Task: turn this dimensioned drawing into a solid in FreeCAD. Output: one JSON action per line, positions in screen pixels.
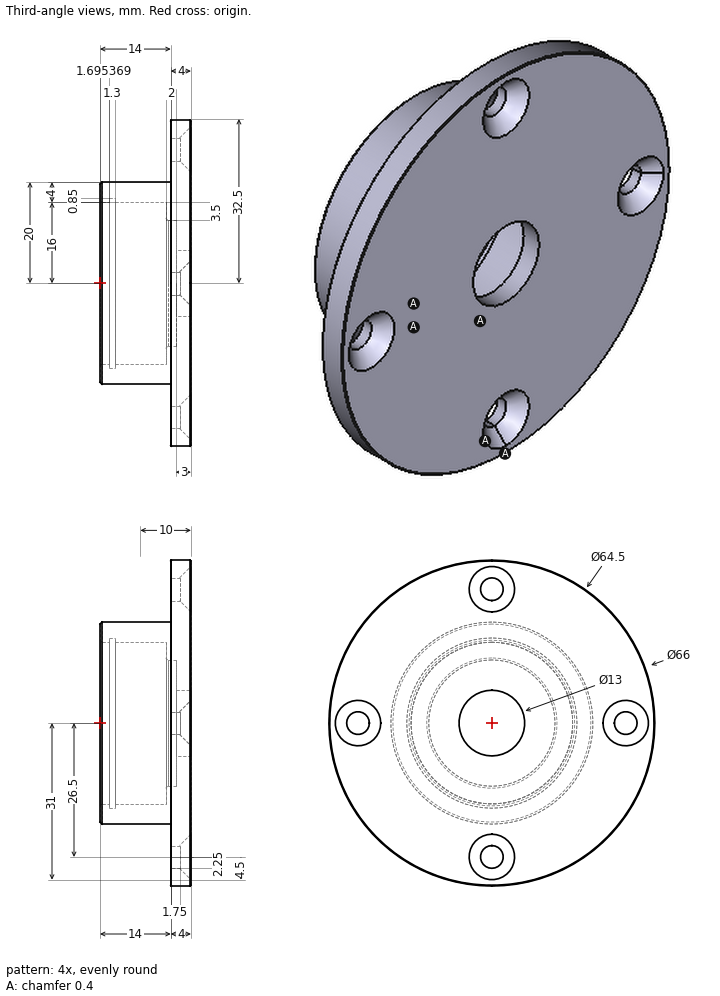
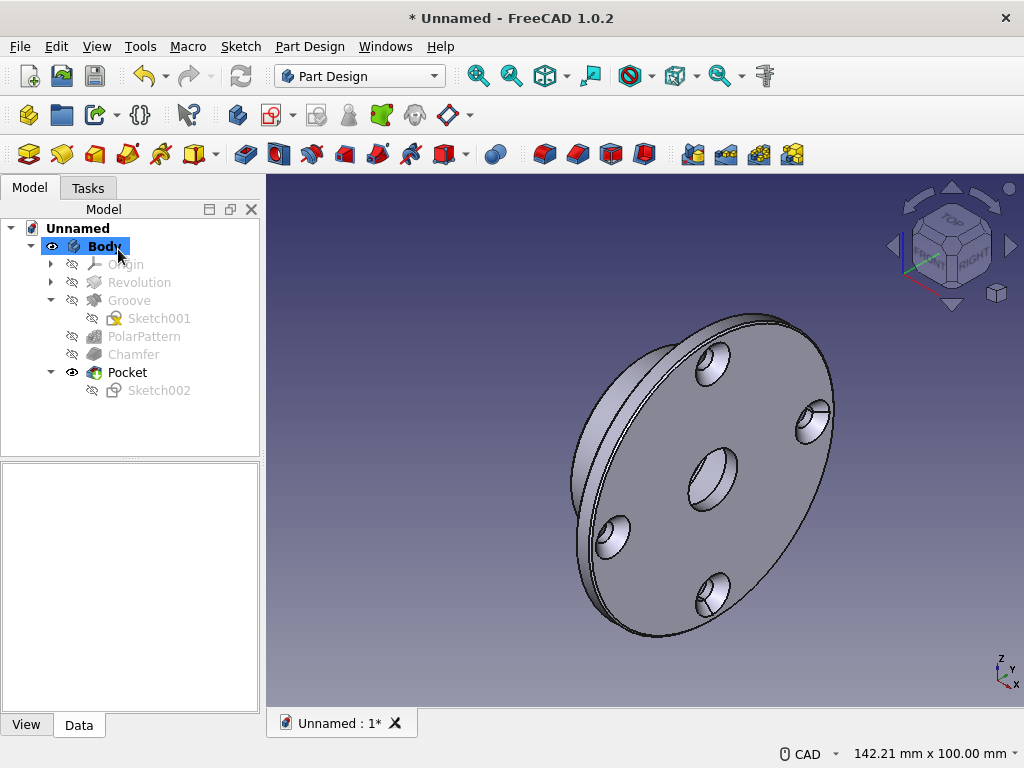
{"action": "left_click", "coordinate": [782, 399]}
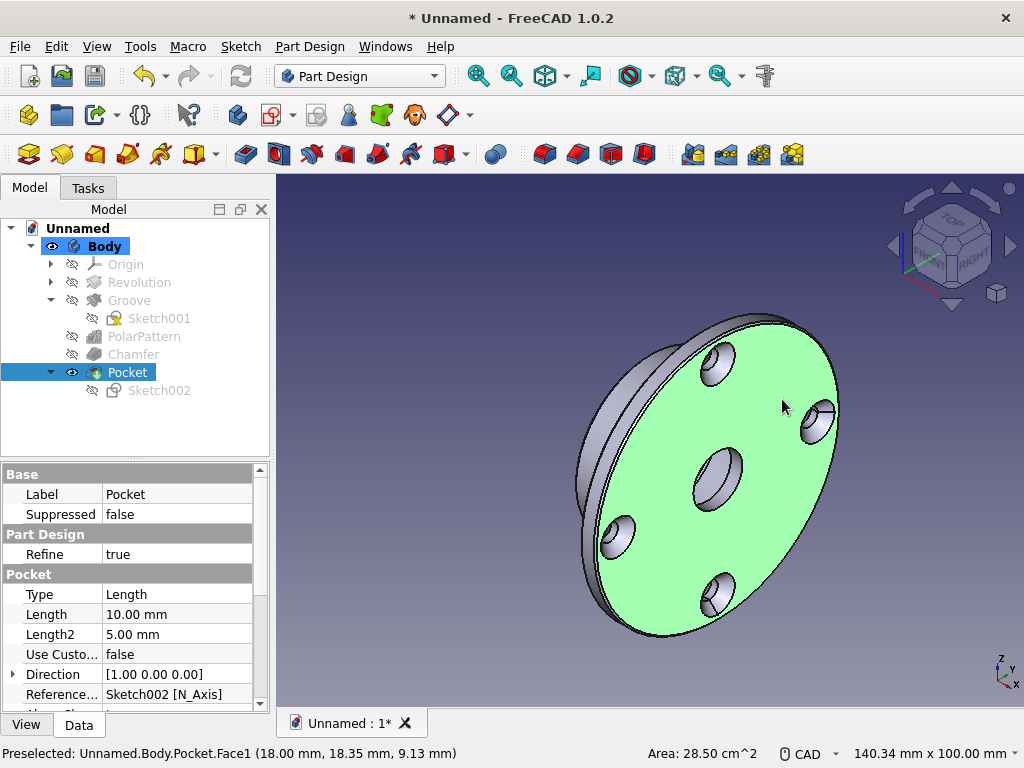
{"action": "left_click", "coordinate": [270, 116]}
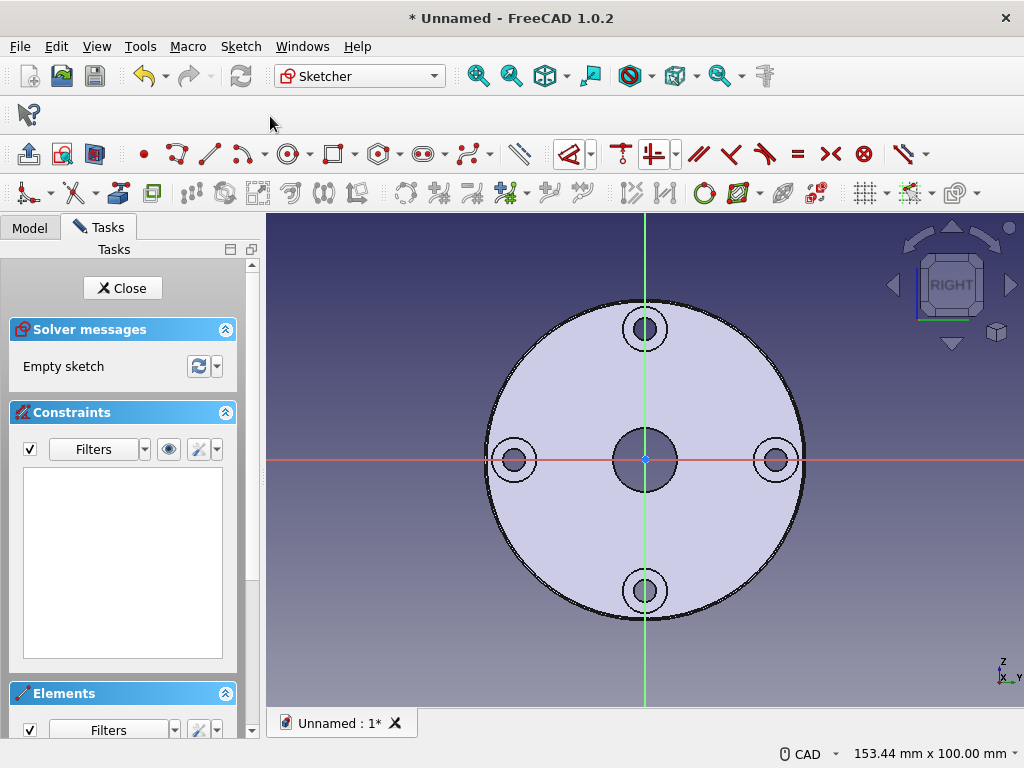
{"action": "left_click", "coordinate": [288, 154]}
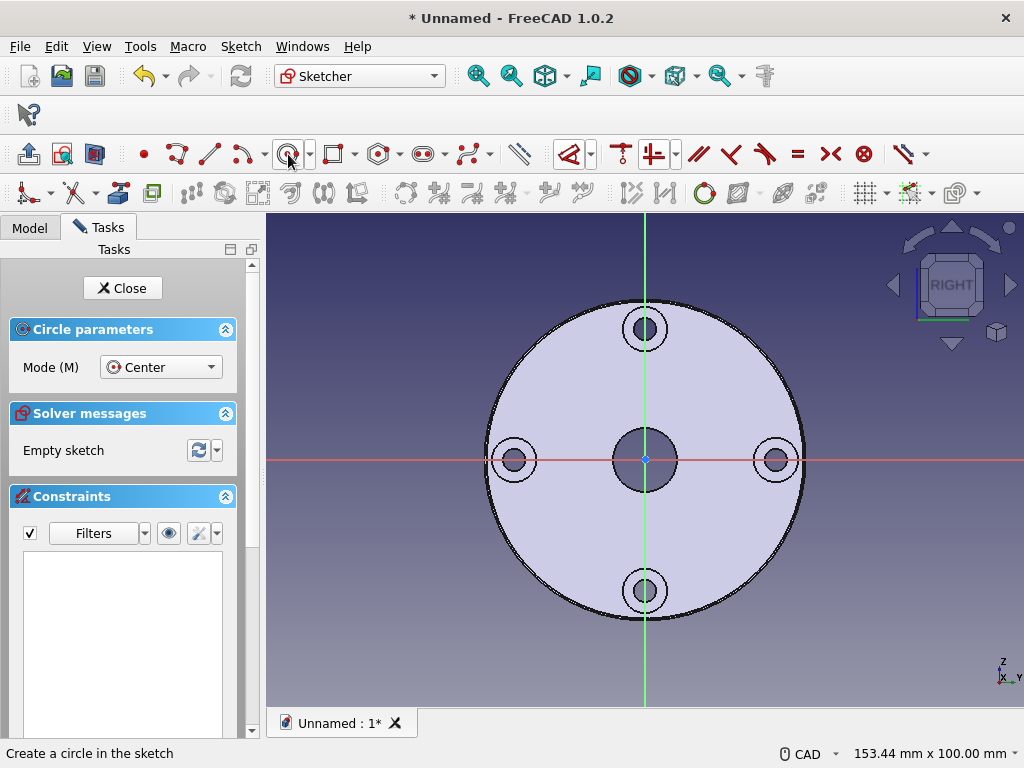
{"action": "left_click", "coordinate": [645, 460]}
{"action": "mouse_move", "coordinate": [760, 345]}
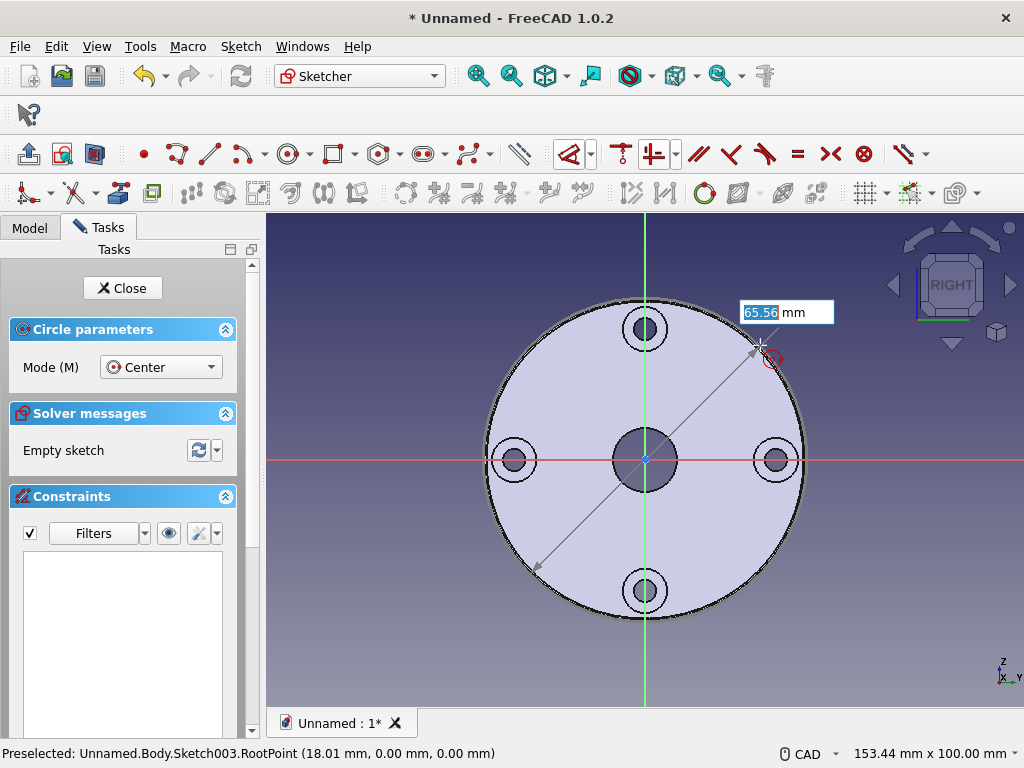
{"action": "type", "text": "66"}
{"action": "key", "text": "Return"}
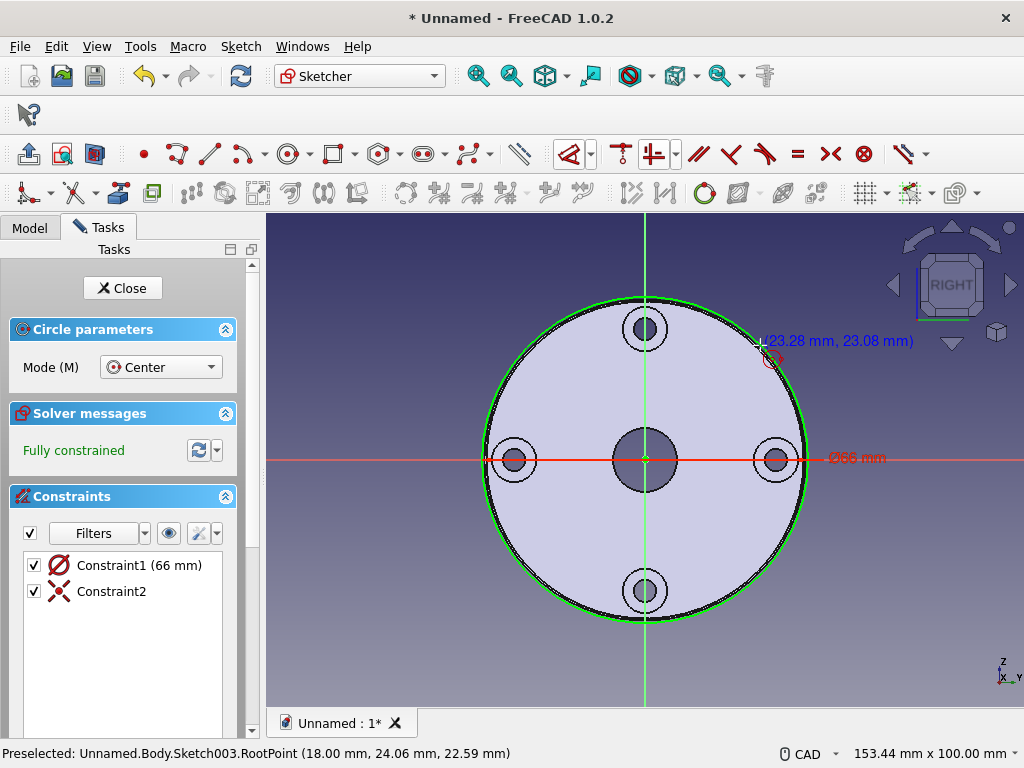
{"action": "left_click", "coordinate": [645, 460]}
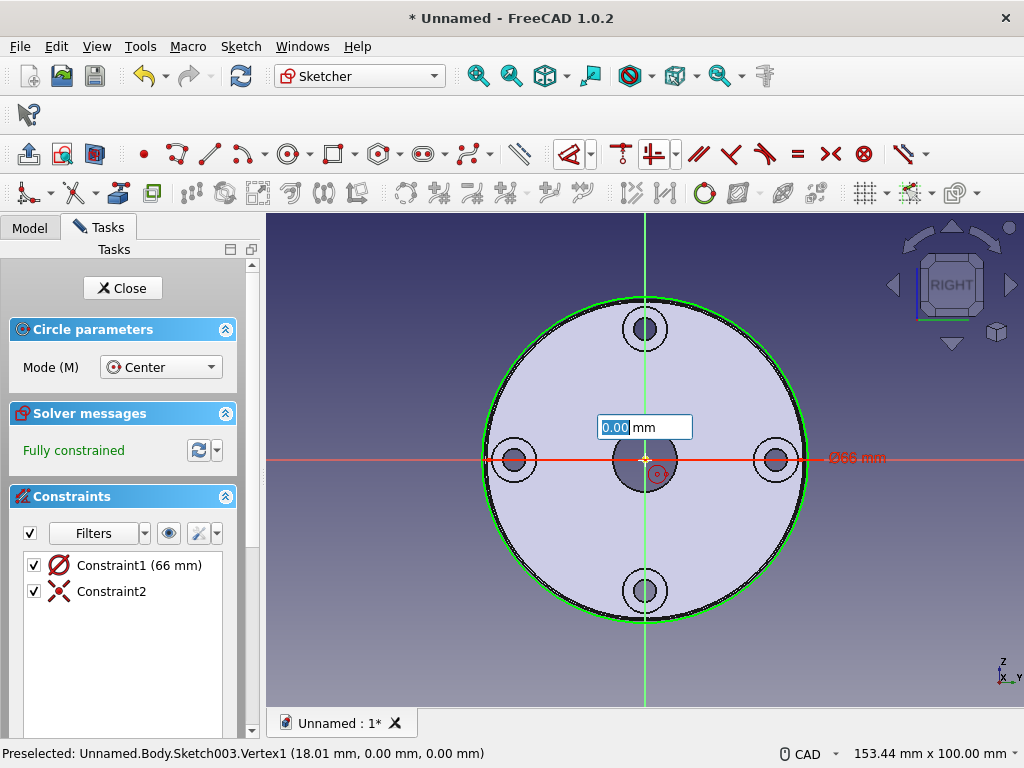
{"action": "scroll", "coordinate": [758, 347], "scroll_direction": "up", "scroll_amount": 8}
{"action": "mouse_move", "coordinate": [754, 348]}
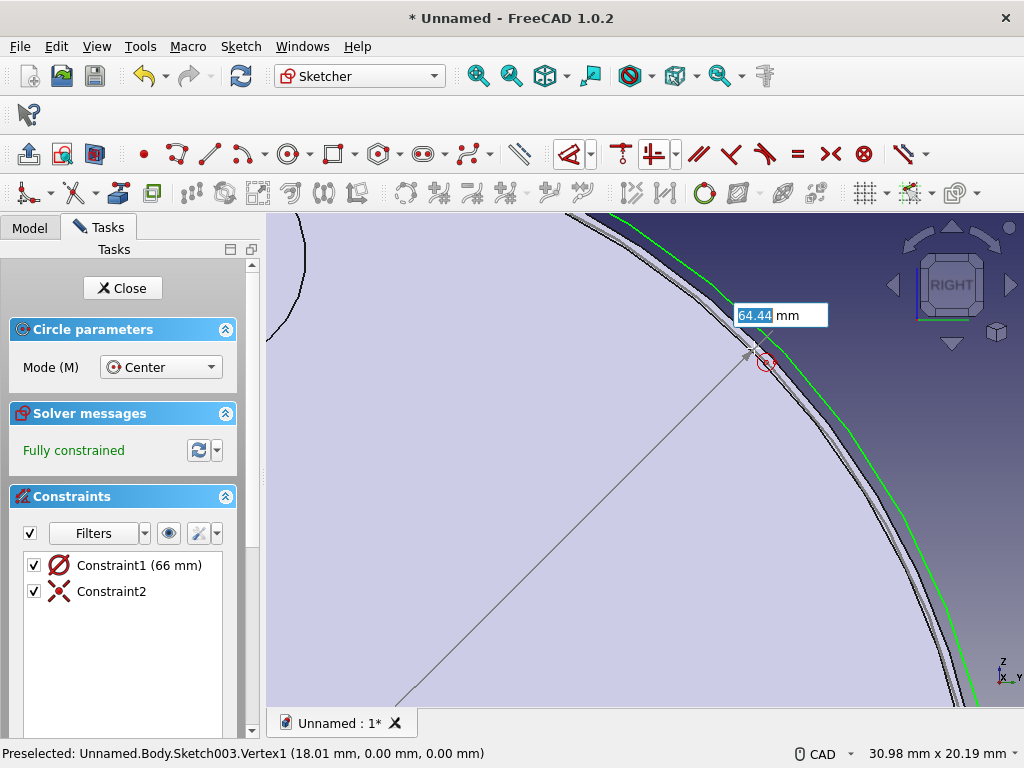
{"action": "type", "text": "64.5"}
{"action": "key", "text": "Return"}
{"action": "key", "text": "Escape"}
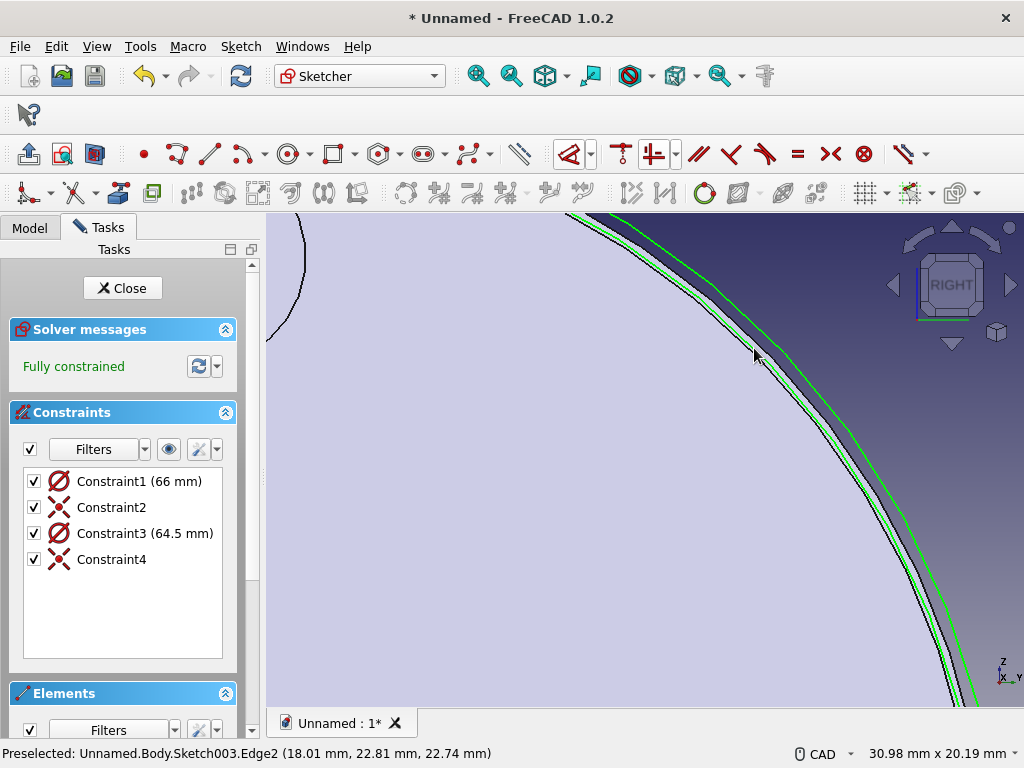
{"action": "left_click", "coordinate": [123, 288]}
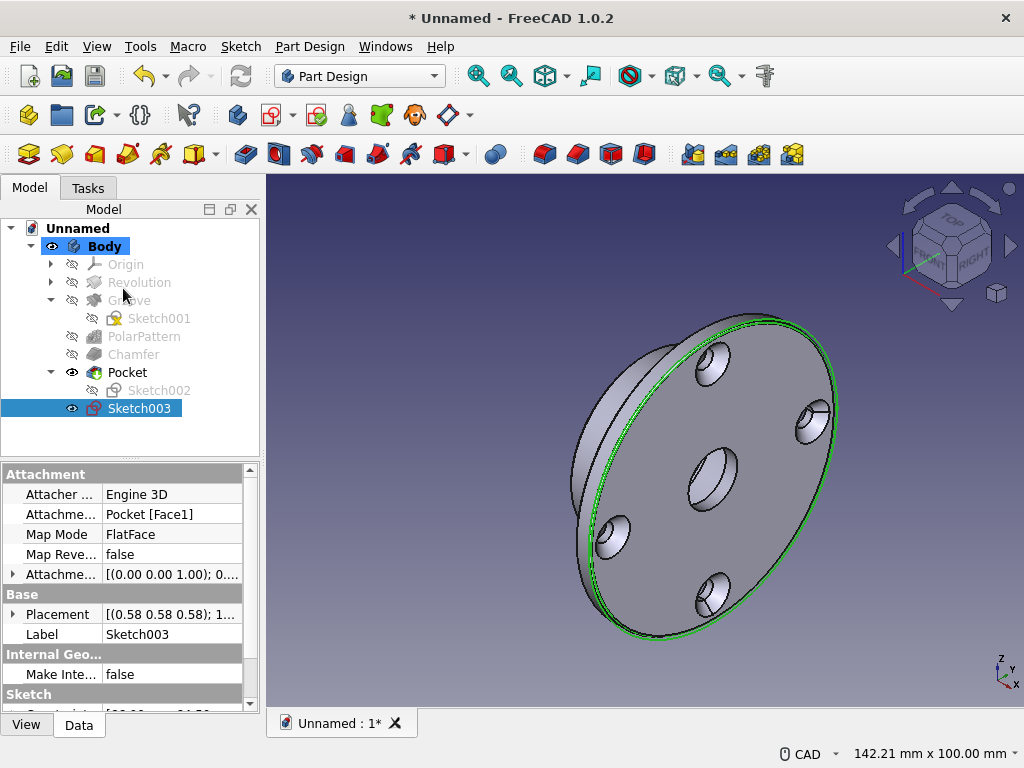
{"action": "left_click", "coordinate": [246, 154]}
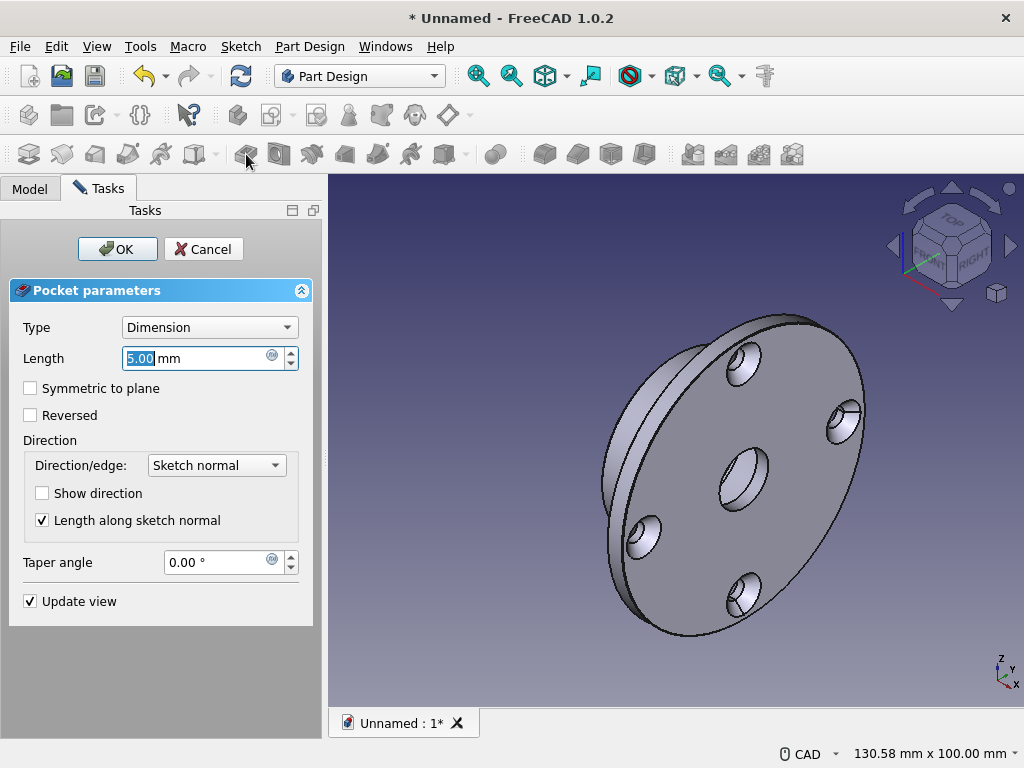
{"action": "type", "text": "10"}
{"action": "key", "text": "Tab"}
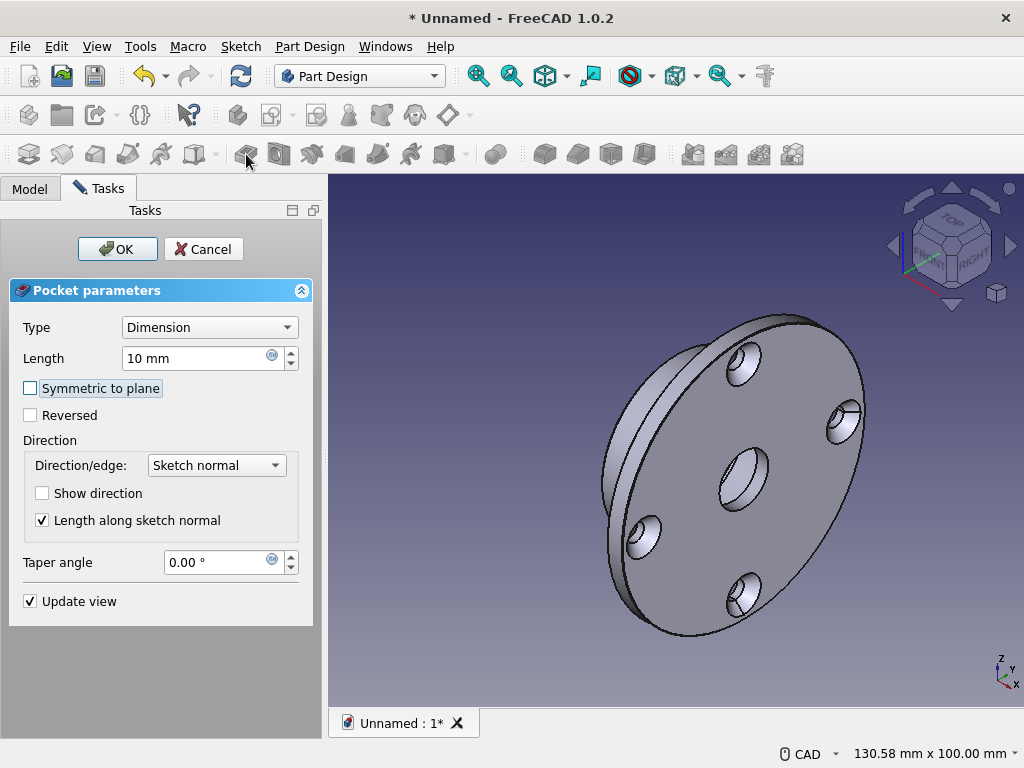
{"action": "left_click", "coordinate": [118, 249]}